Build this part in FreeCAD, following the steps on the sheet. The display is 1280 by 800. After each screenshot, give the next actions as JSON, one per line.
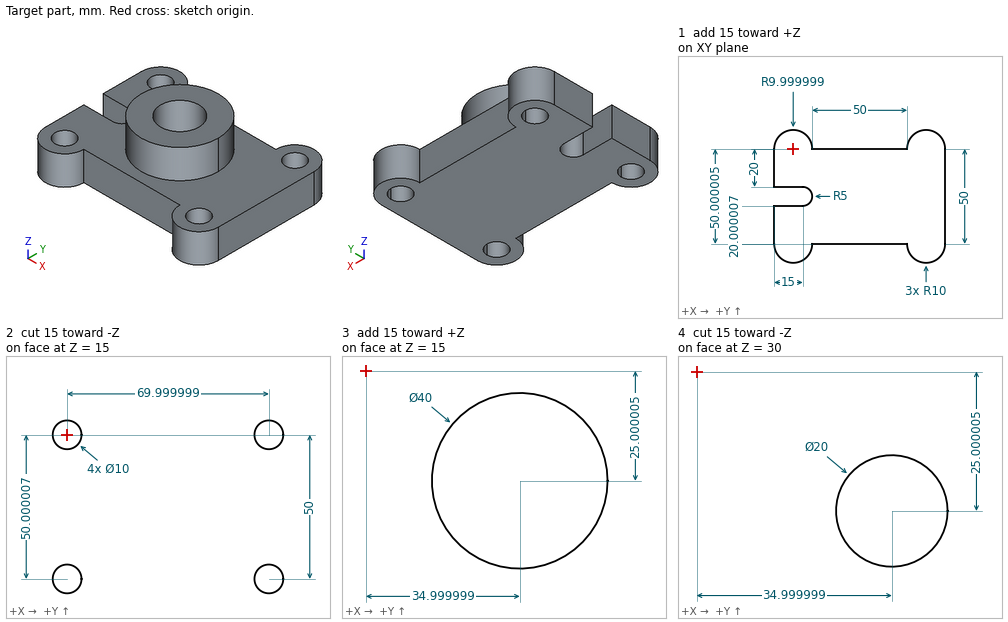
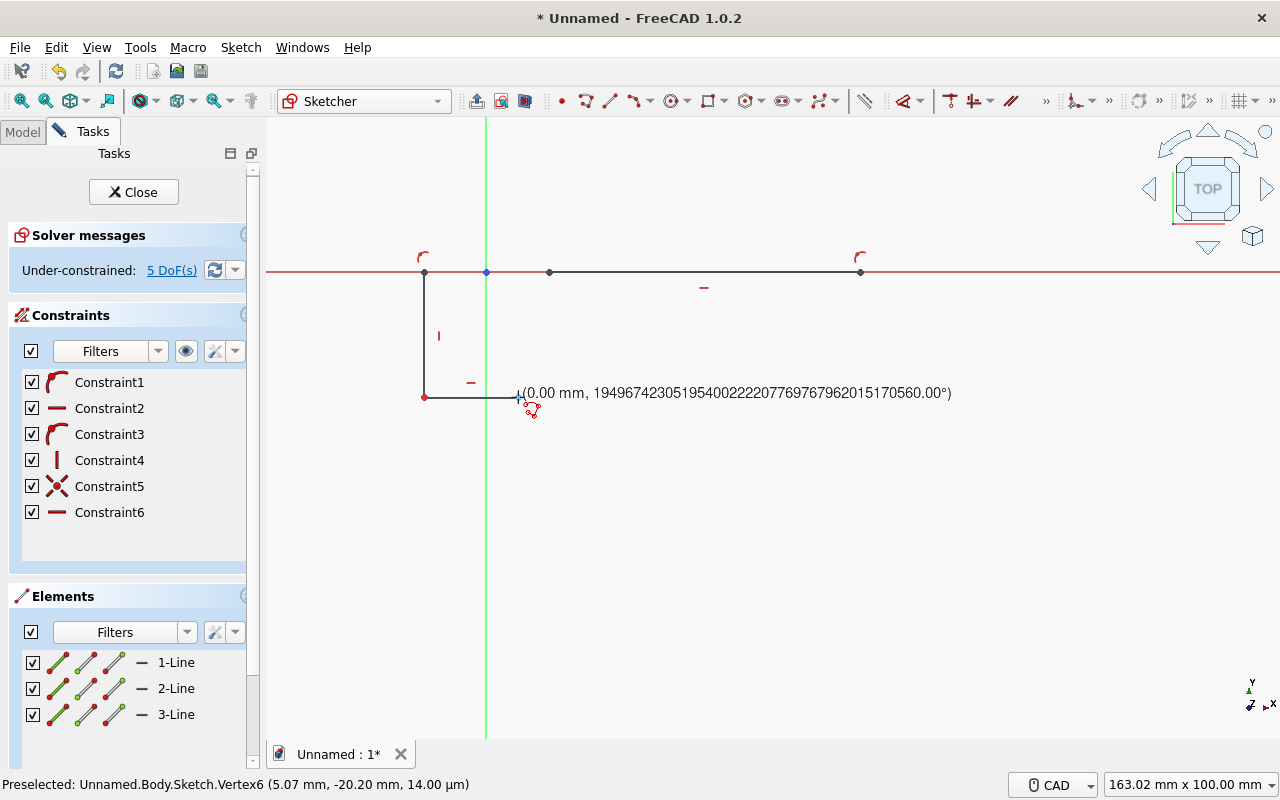
{"action": "left_click", "coordinate": [518, 459]}
{"action": "left_click", "coordinate": [424, 459]}
{"action": "left_click", "coordinate": [424, 583]}
{"action": "right_click", "coordinate": [424, 583]}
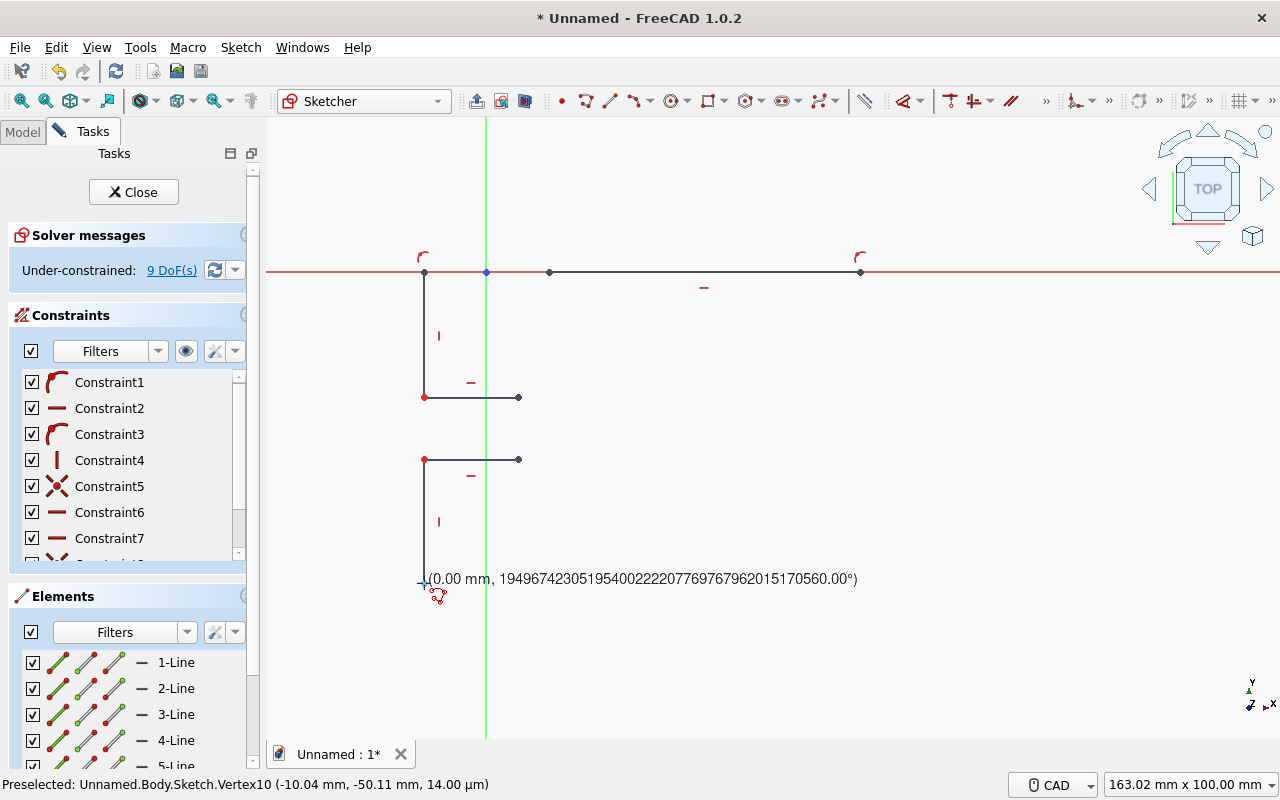
{"action": "left_click", "coordinate": [610, 102]}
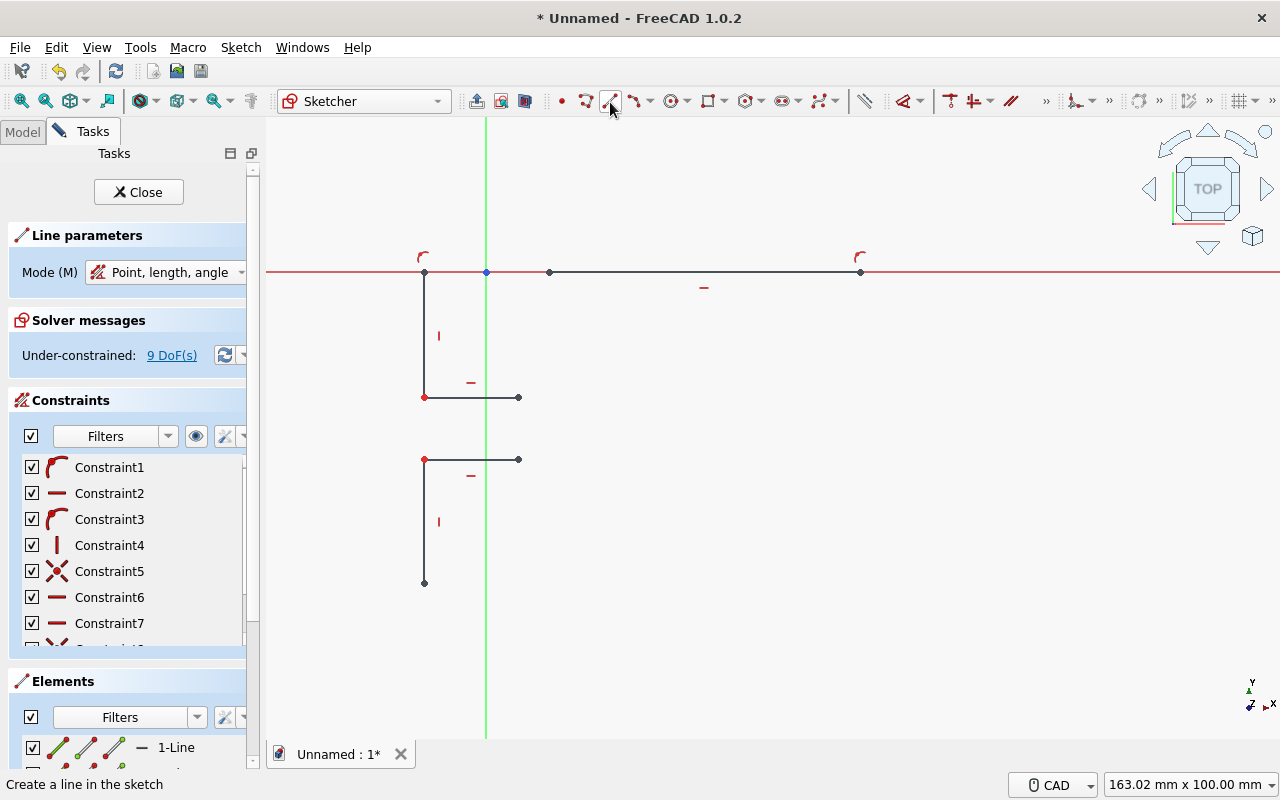
{"action": "left_click", "coordinate": [549, 583]}
{"action": "left_click", "coordinate": [860, 583]}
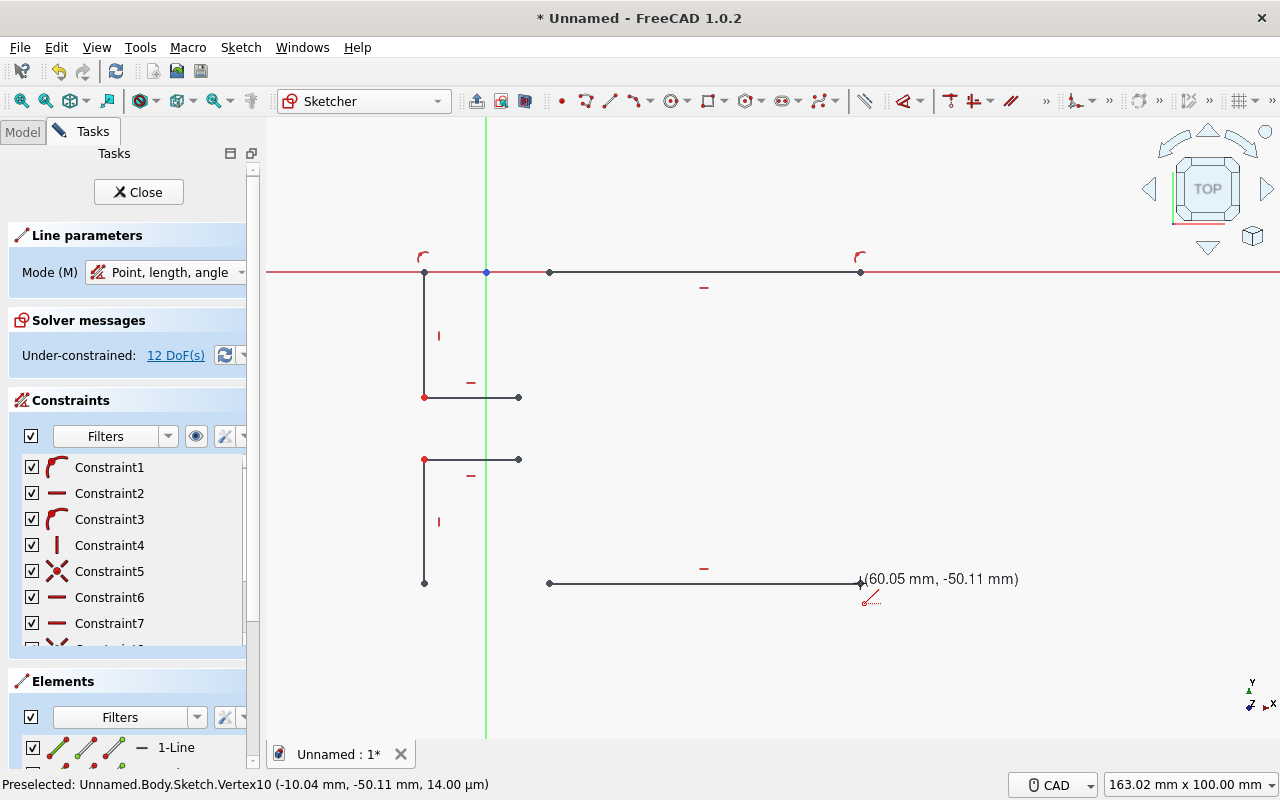
{"action": "left_click", "coordinate": [984, 583]}
{"action": "left_click", "coordinate": [984, 272]}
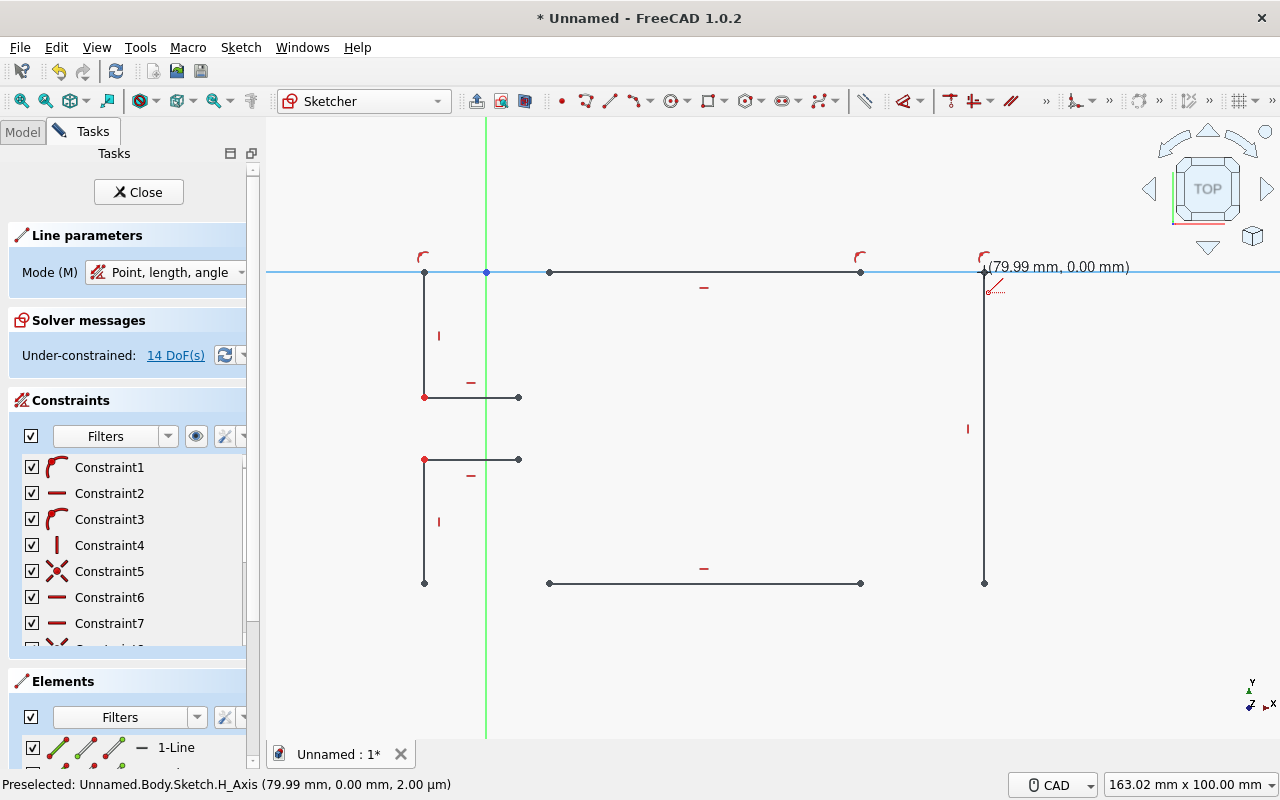
{"action": "left_click", "coordinate": [634, 102]}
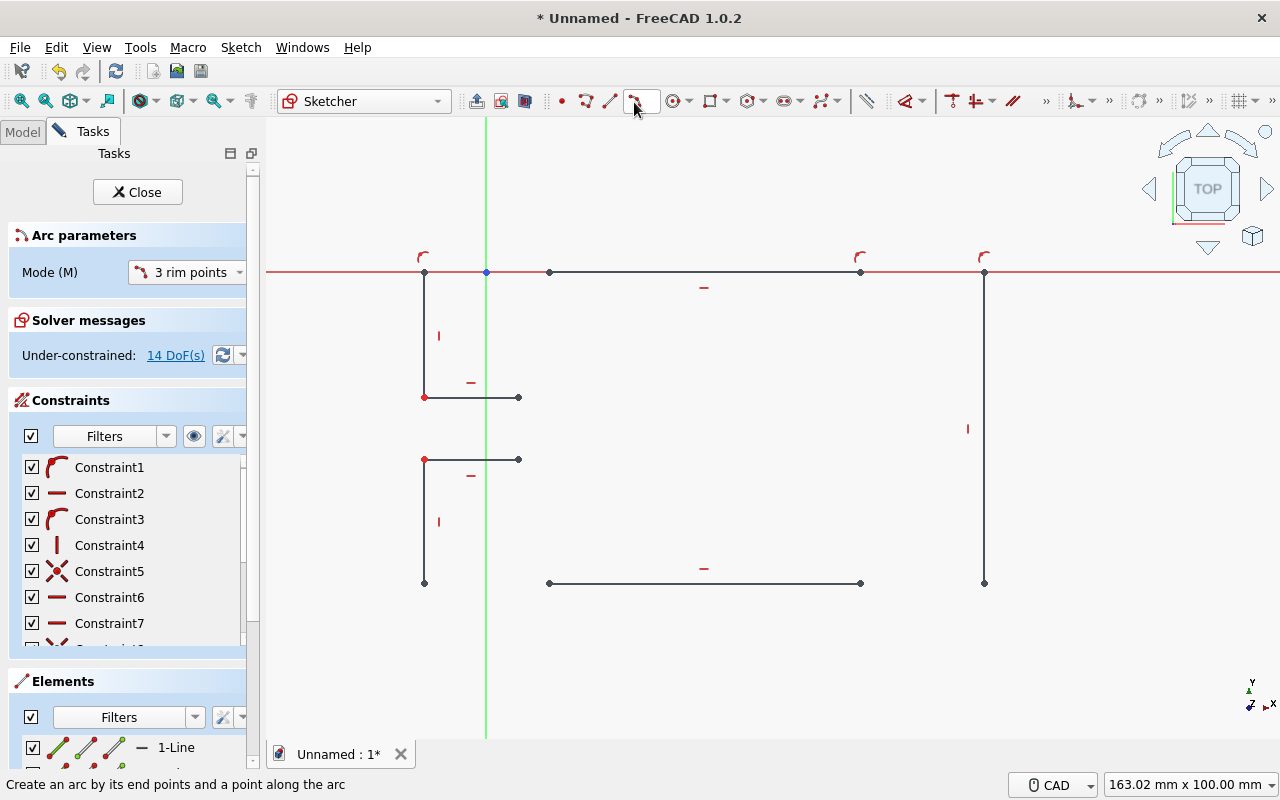
{"action": "left_click", "coordinate": [549, 272]}
{"action": "left_click", "coordinate": [424, 272]}
{"action": "left_click", "coordinate": [506, 213]}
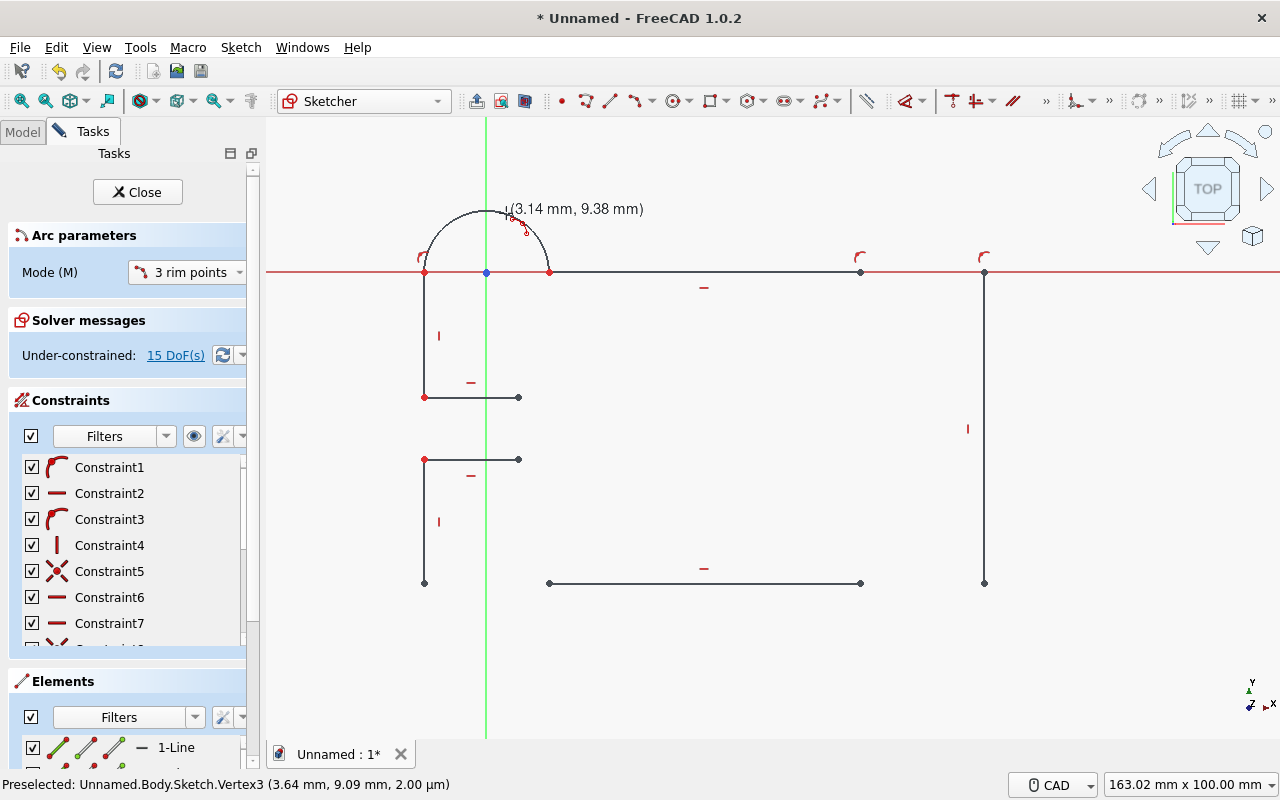
{"action": "left_click", "coordinate": [518, 398]}
{"action": "left_click", "coordinate": [518, 460]}
{"action": "left_click", "coordinate": [549, 428]}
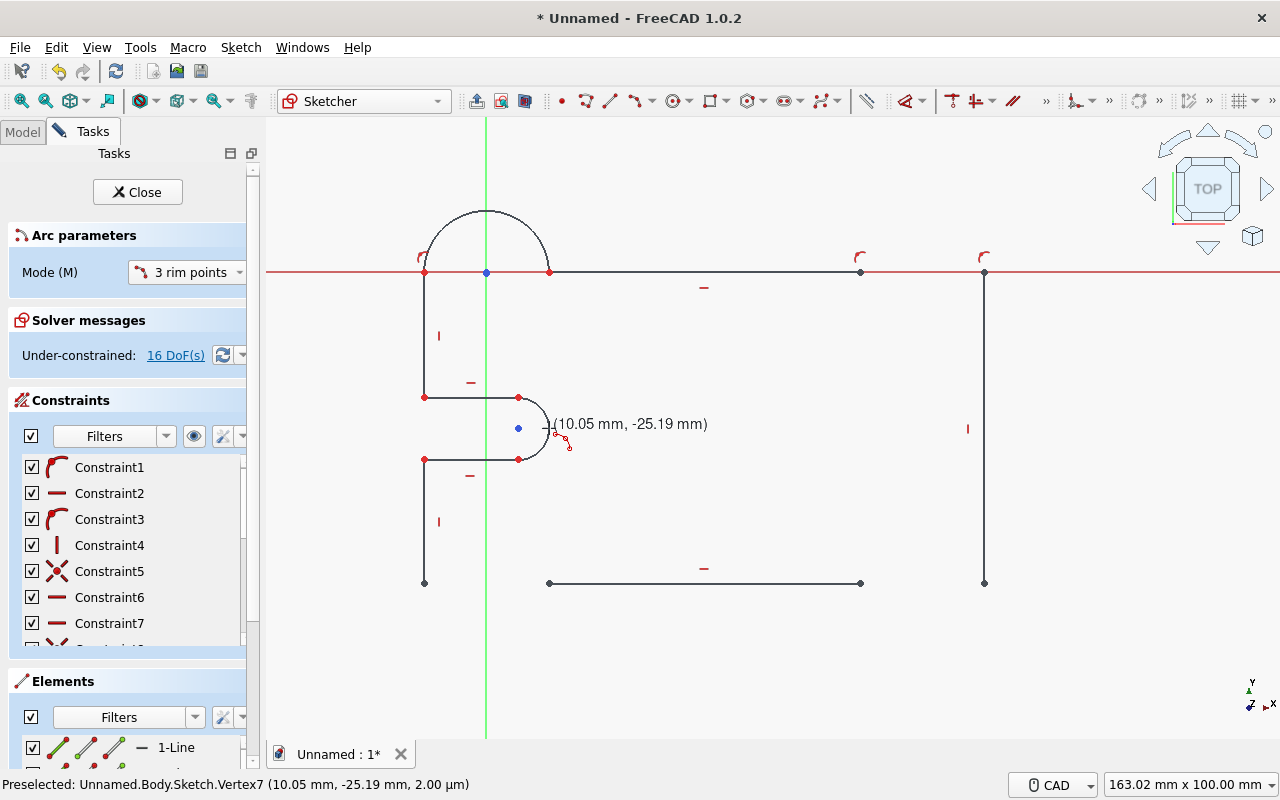
{"action": "left_click", "coordinate": [424, 584]}
{"action": "left_click", "coordinate": [549, 584]}
{"action": "left_click", "coordinate": [467, 642]}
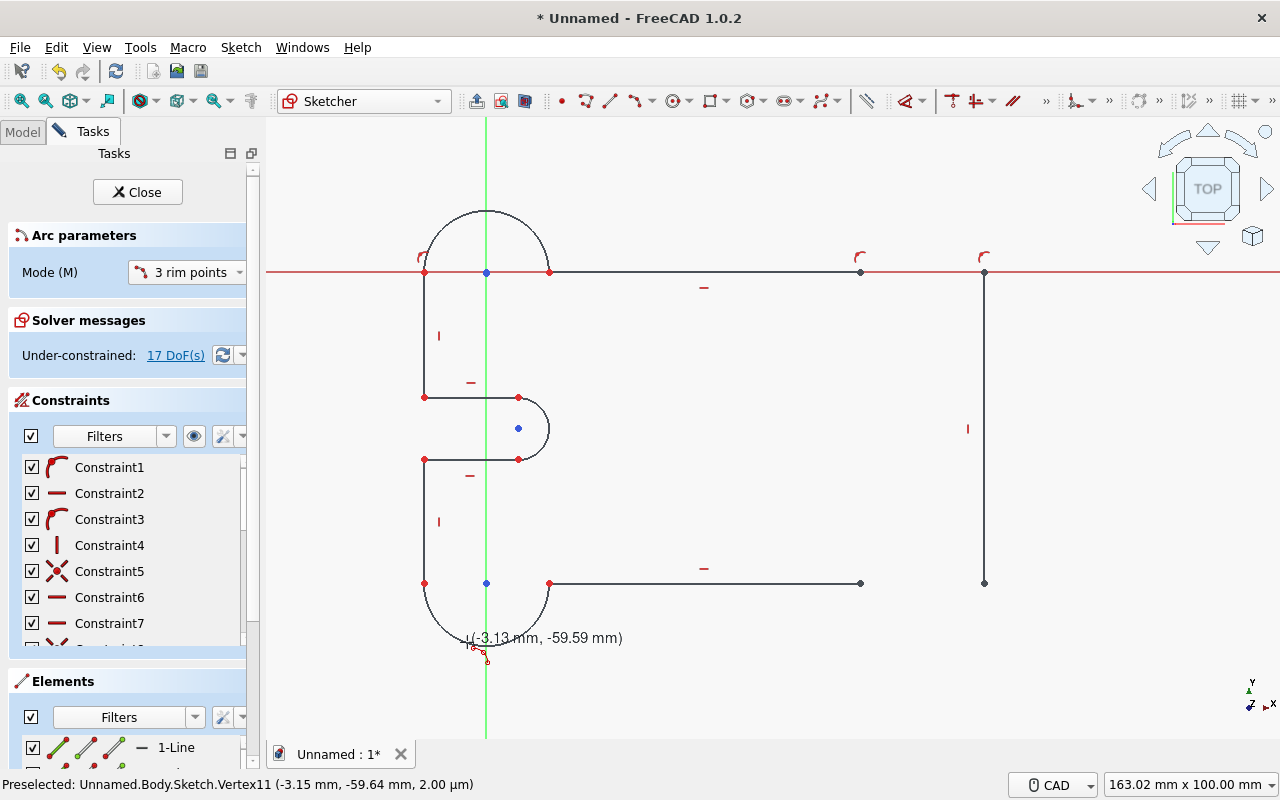
{"action": "left_click", "coordinate": [860, 584]}
{"action": "left_click", "coordinate": [984, 584]}
{"action": "left_click", "coordinate": [922, 646]}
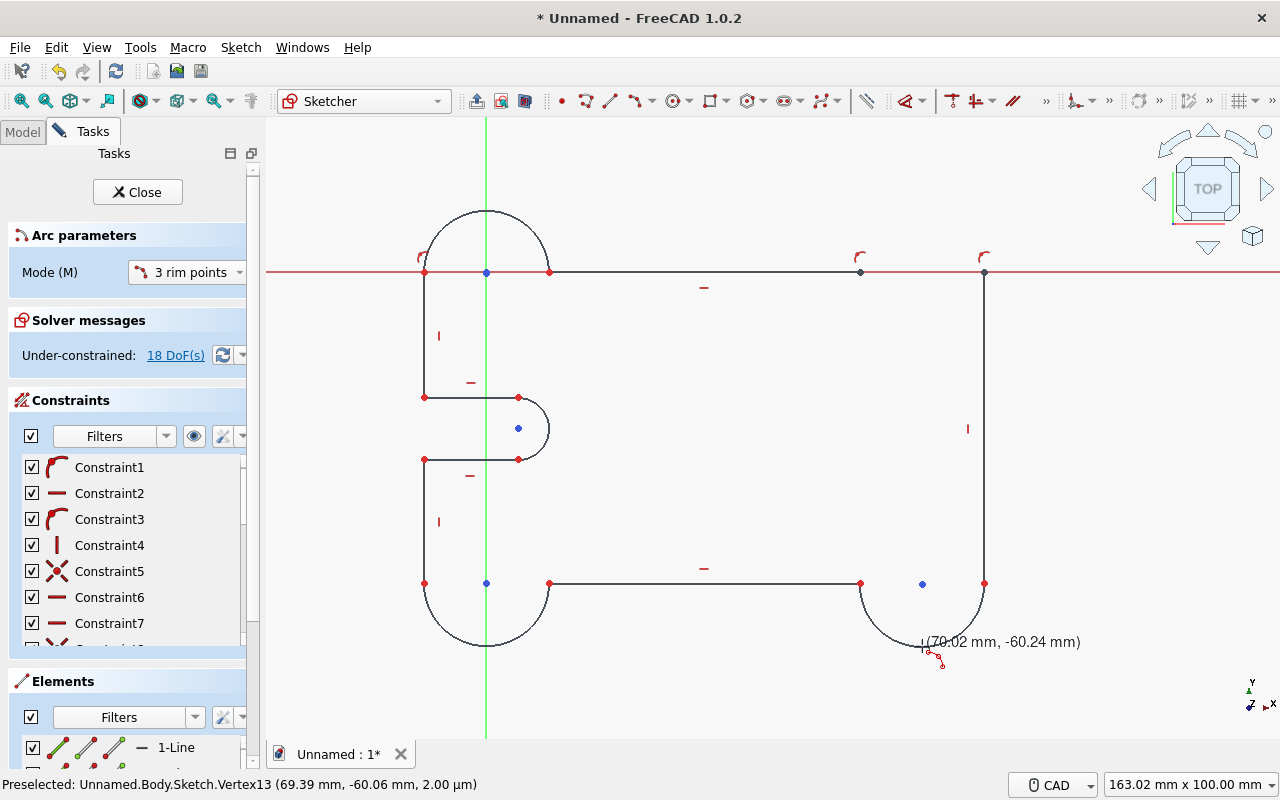
{"action": "left_click", "coordinate": [984, 272]}
{"action": "left_click", "coordinate": [860, 272]}
{"action": "left_click", "coordinate": [922, 210]}
{"action": "key", "text": "Escape"}